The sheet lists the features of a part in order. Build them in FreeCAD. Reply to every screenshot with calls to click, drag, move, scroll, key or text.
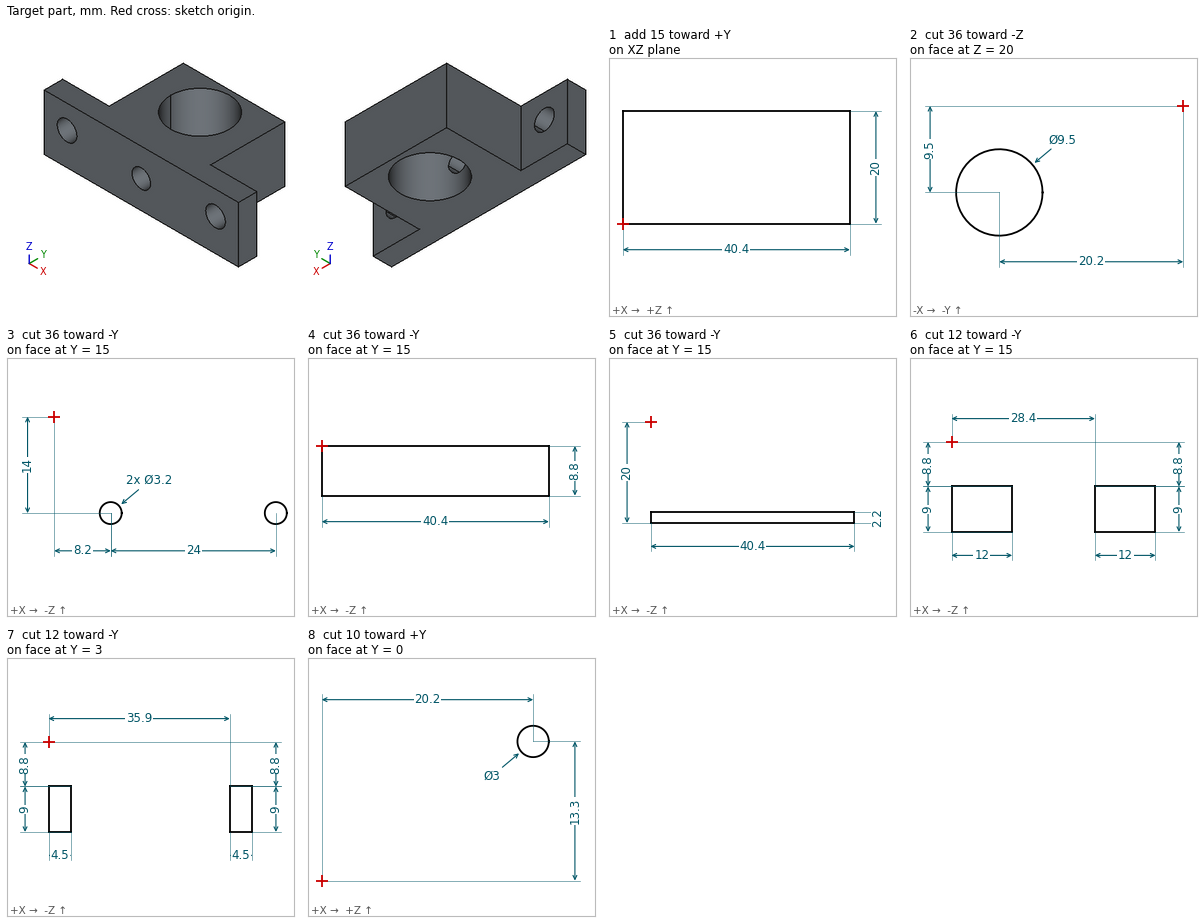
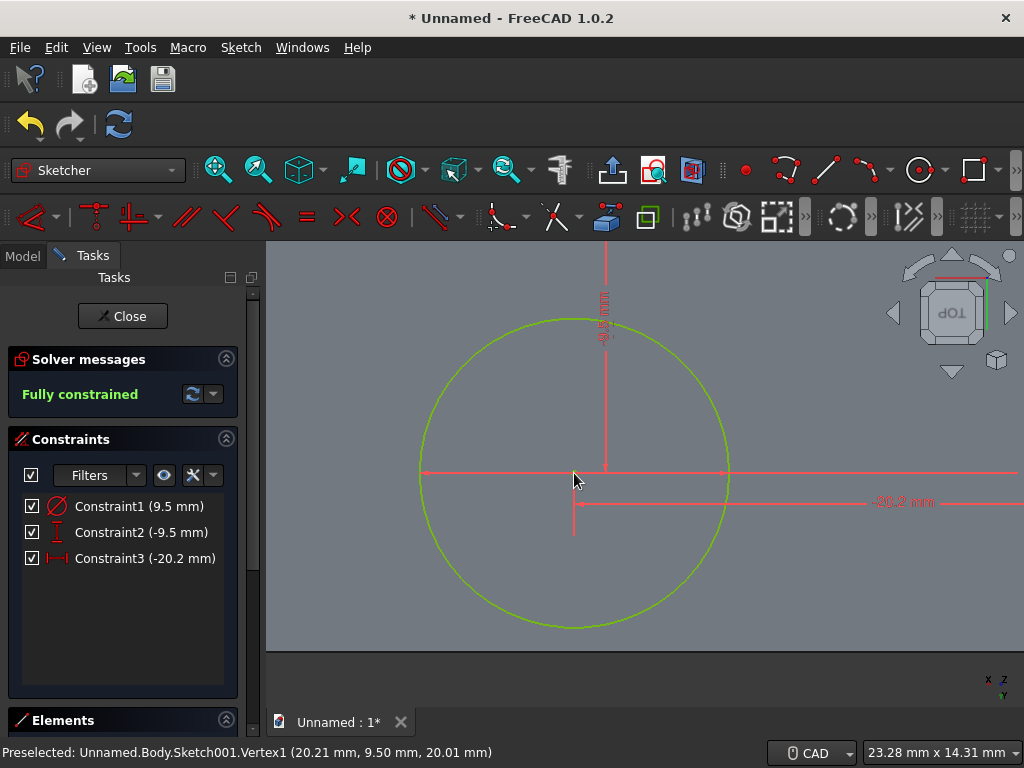
click(123, 316)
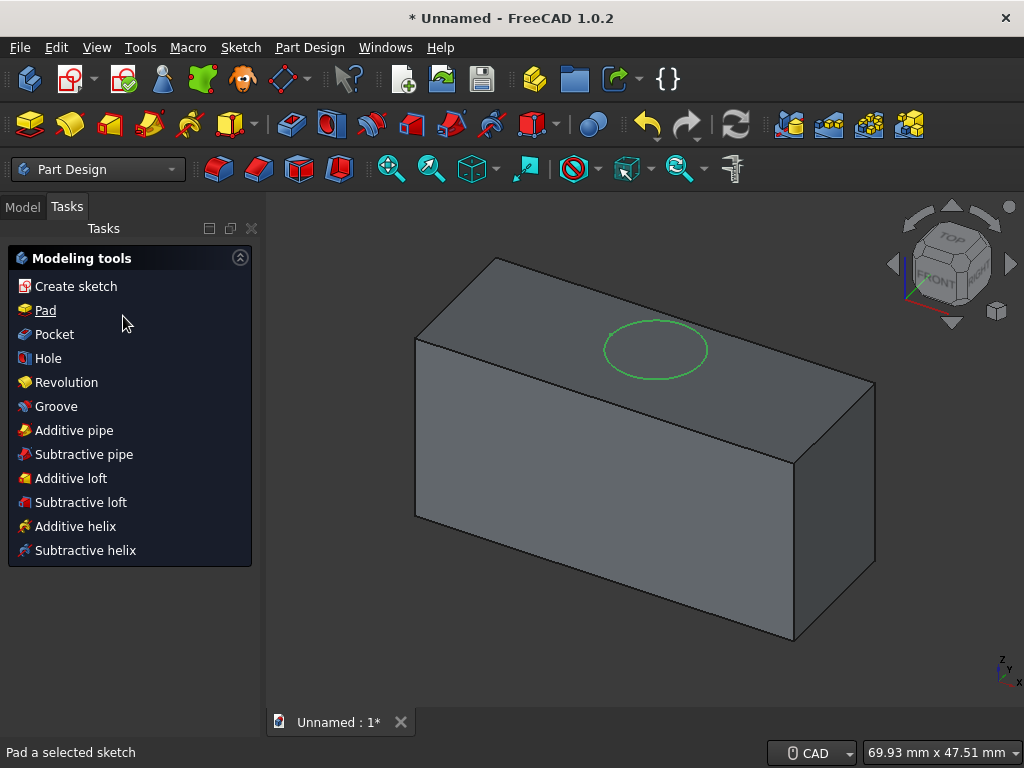
click(292, 124)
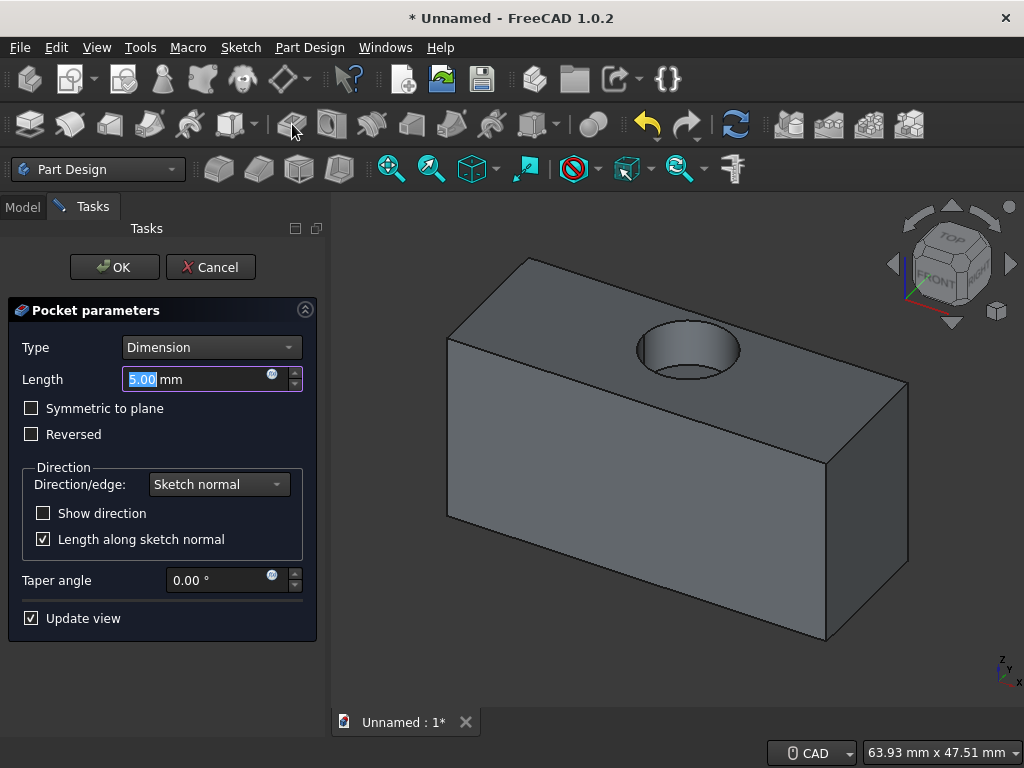
text(36)
key(Tab)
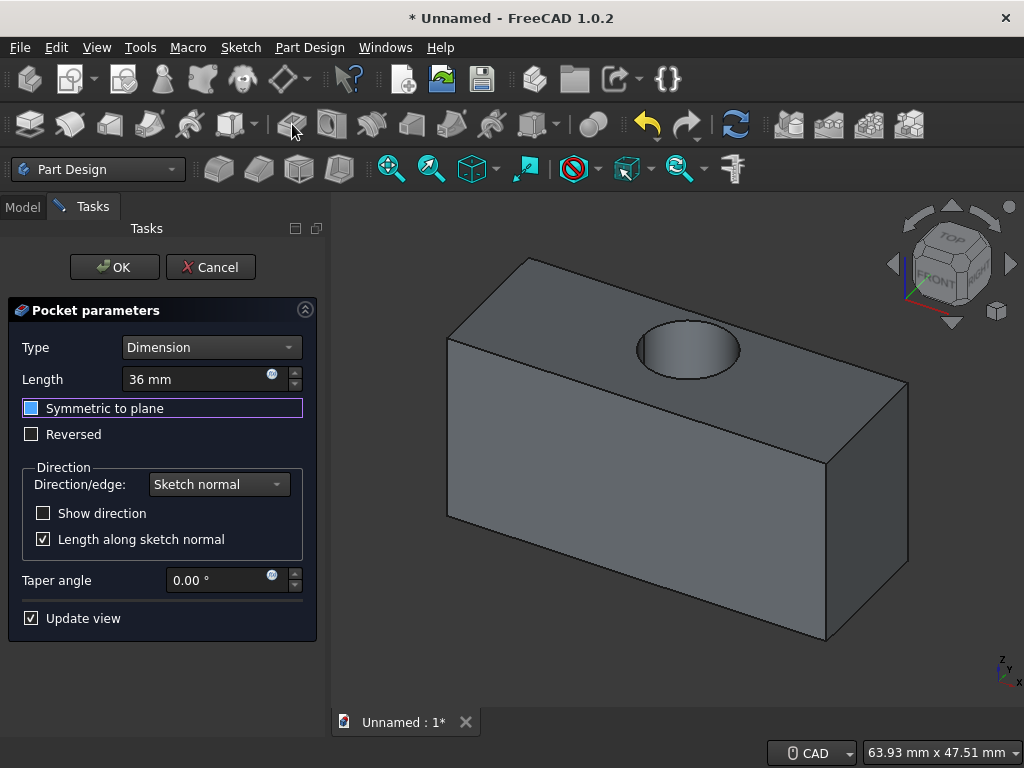
click(115, 267)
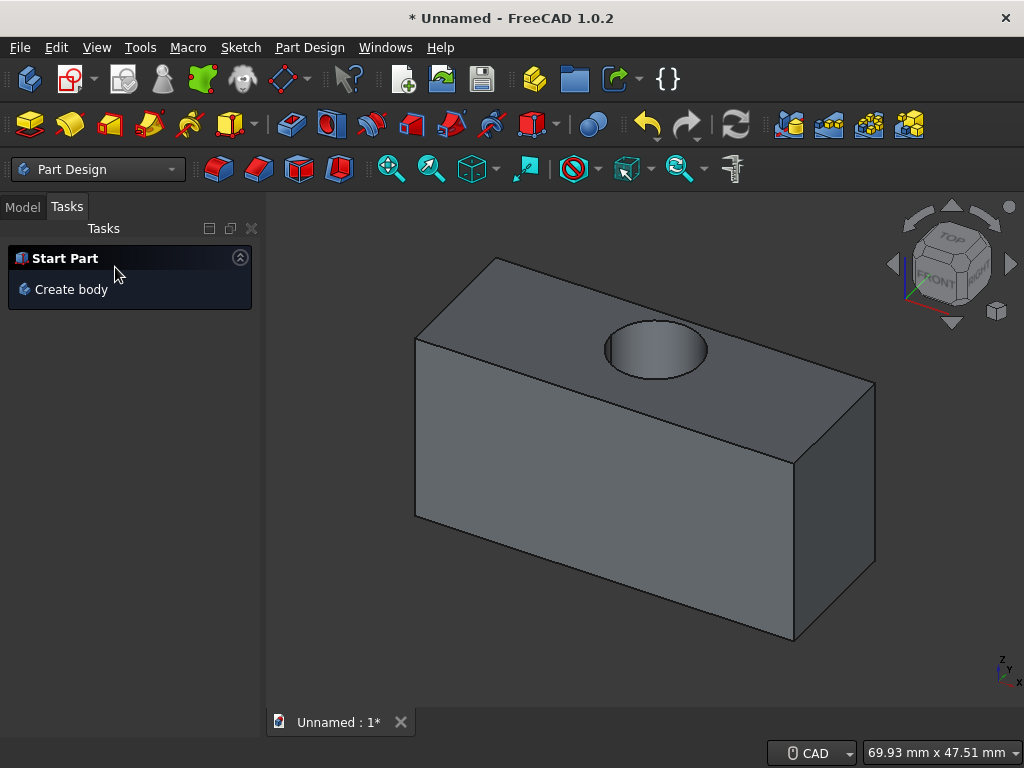
key(4)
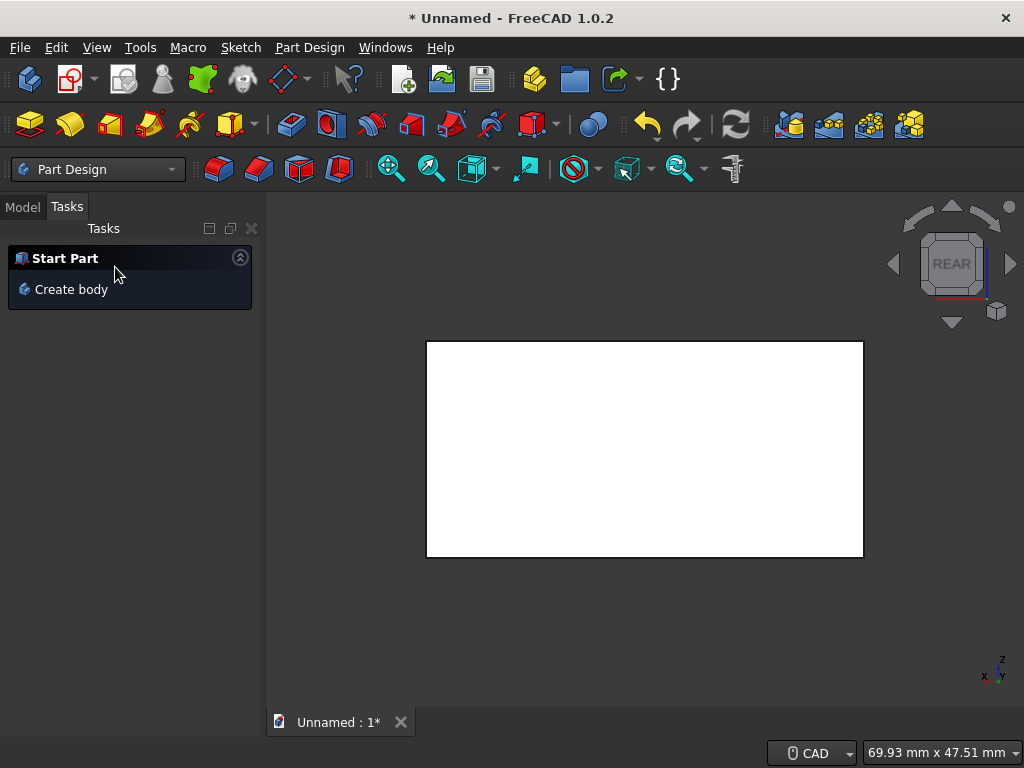
click(582, 449)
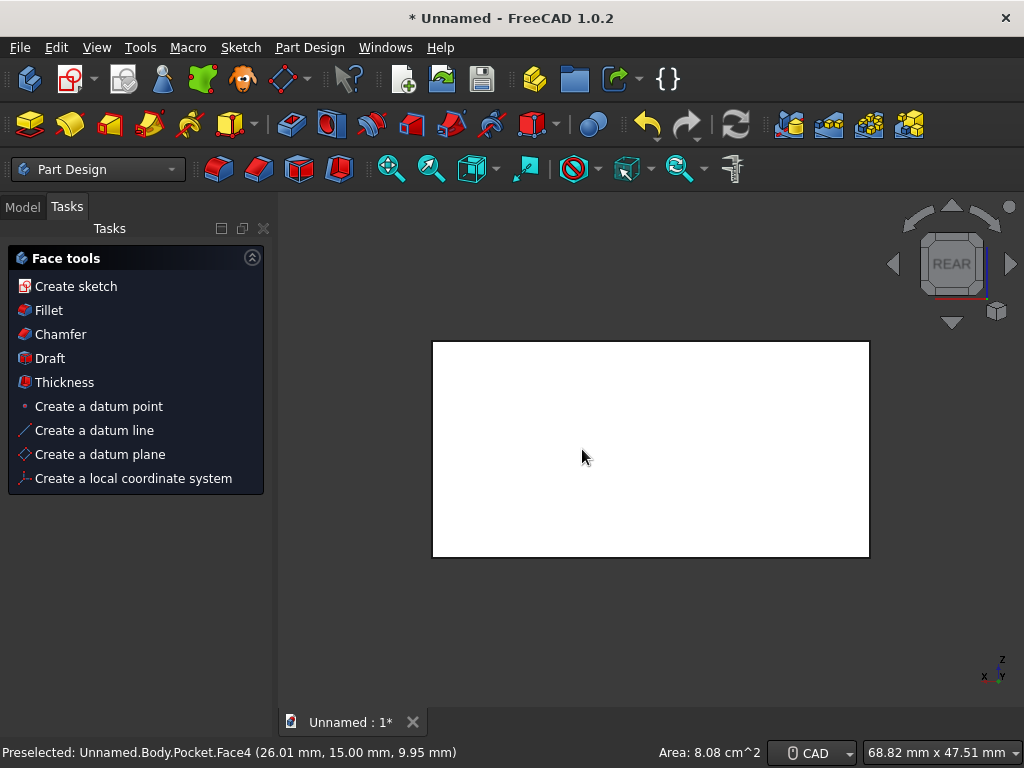
click(70, 80)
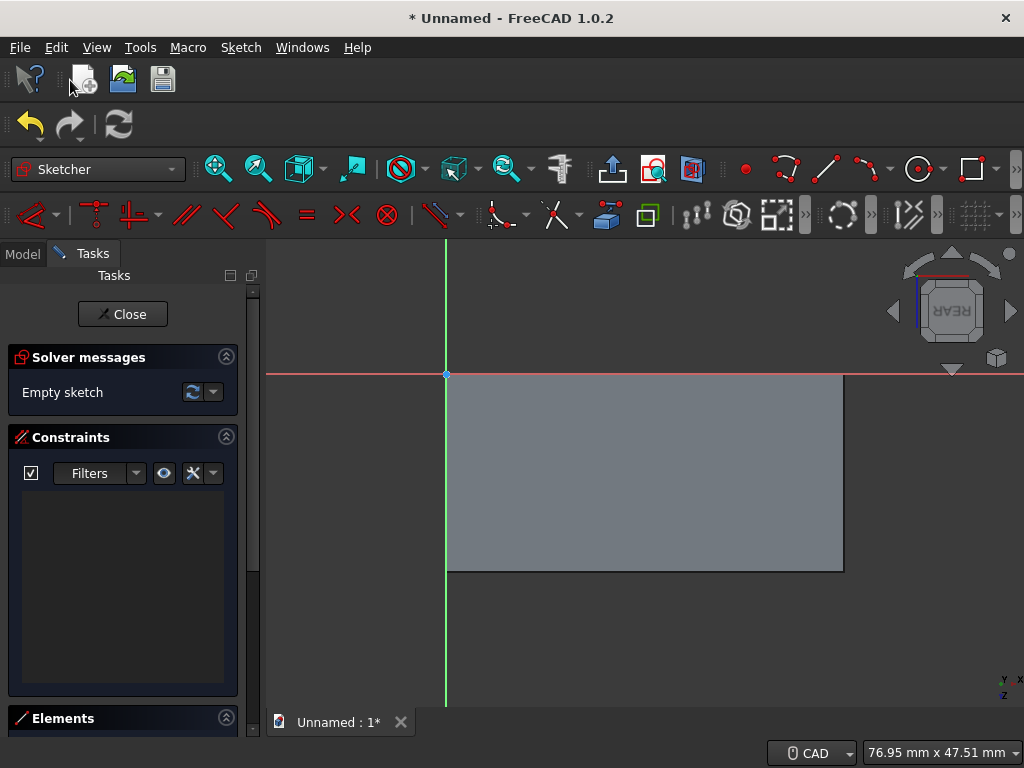
click(920, 170)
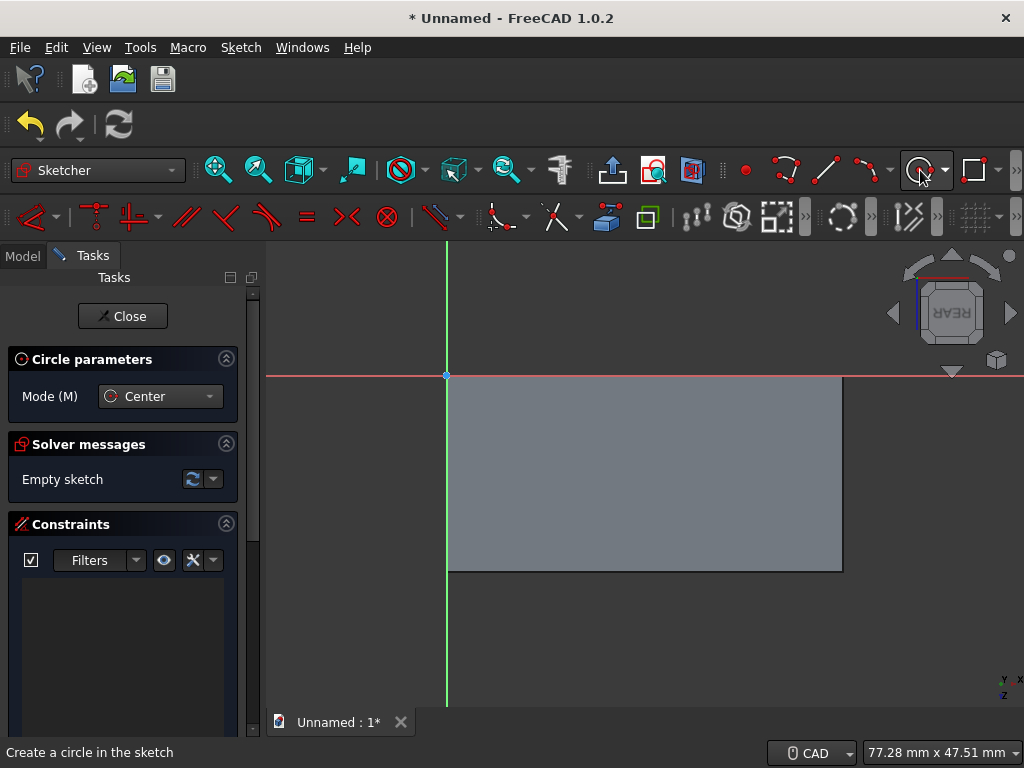
scroll(527, 513, up, 2)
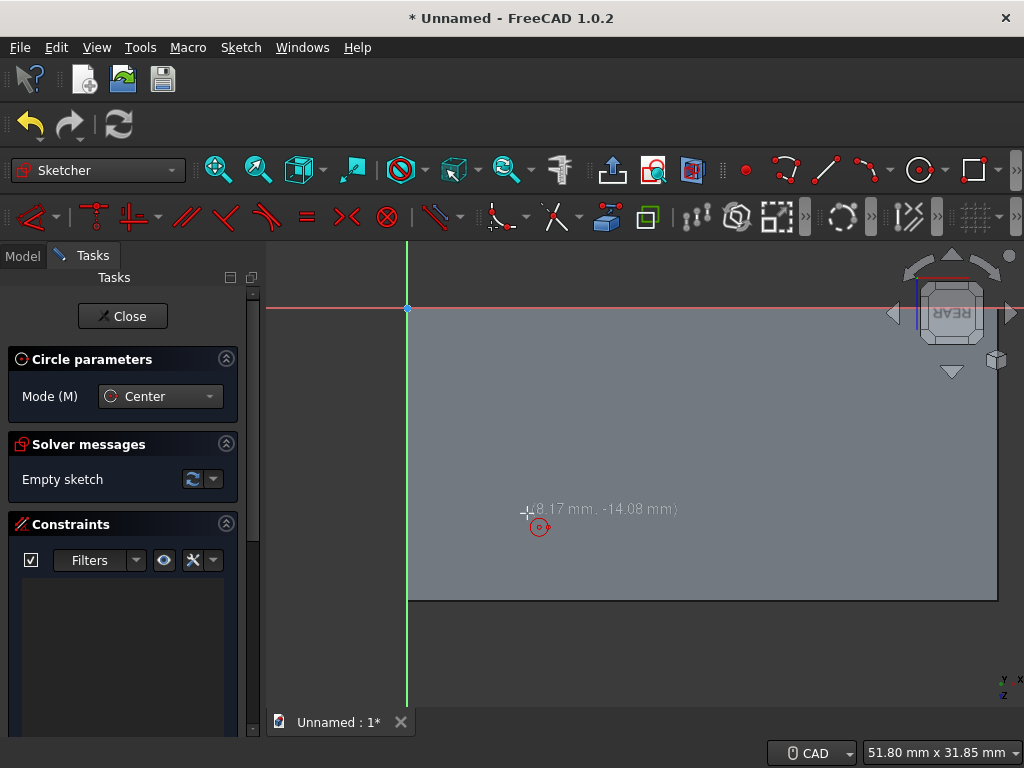
click(527, 513)
move(544, 497)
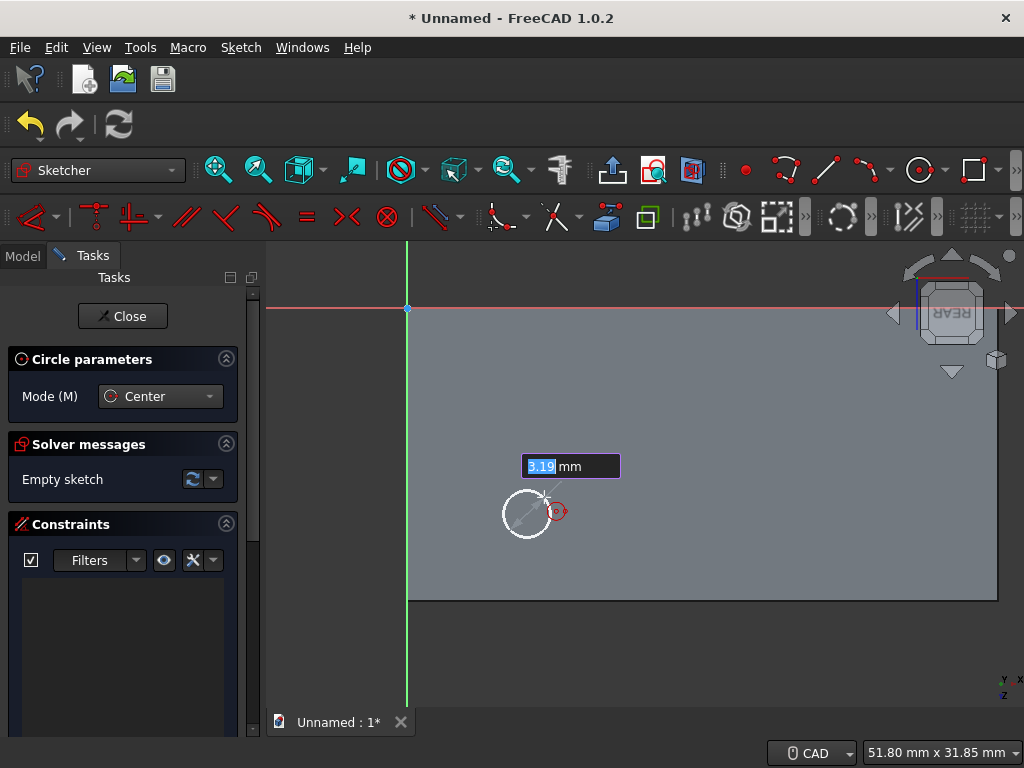
text(3.2)
key(Return)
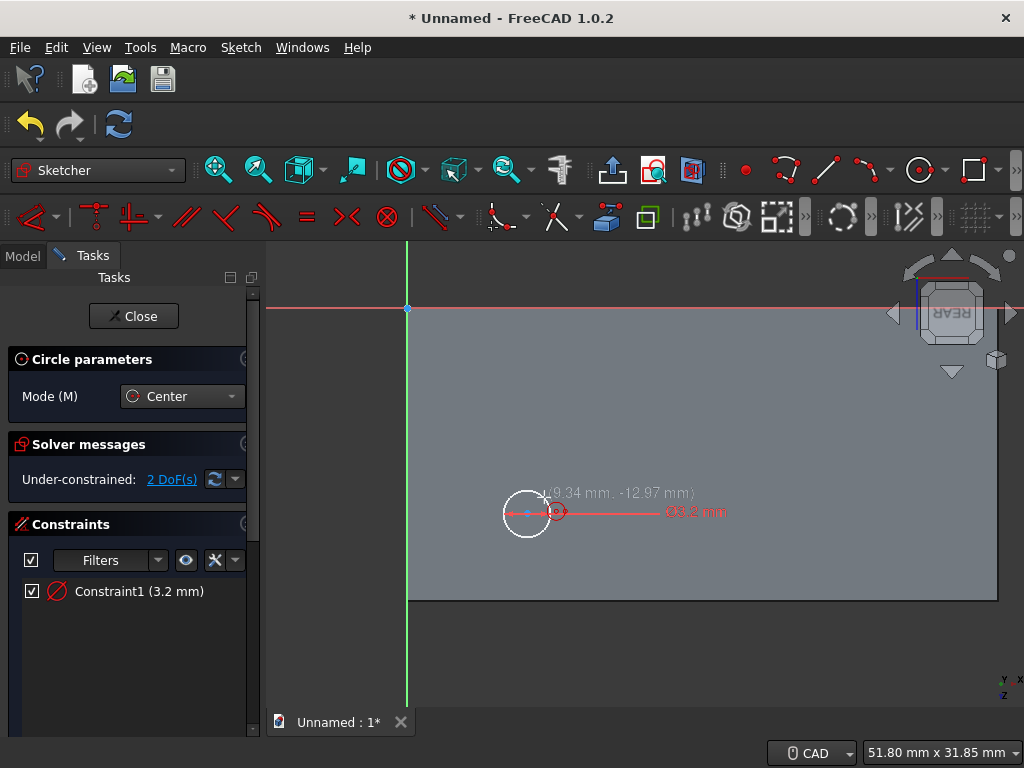
scroll(294, 679, down, 1)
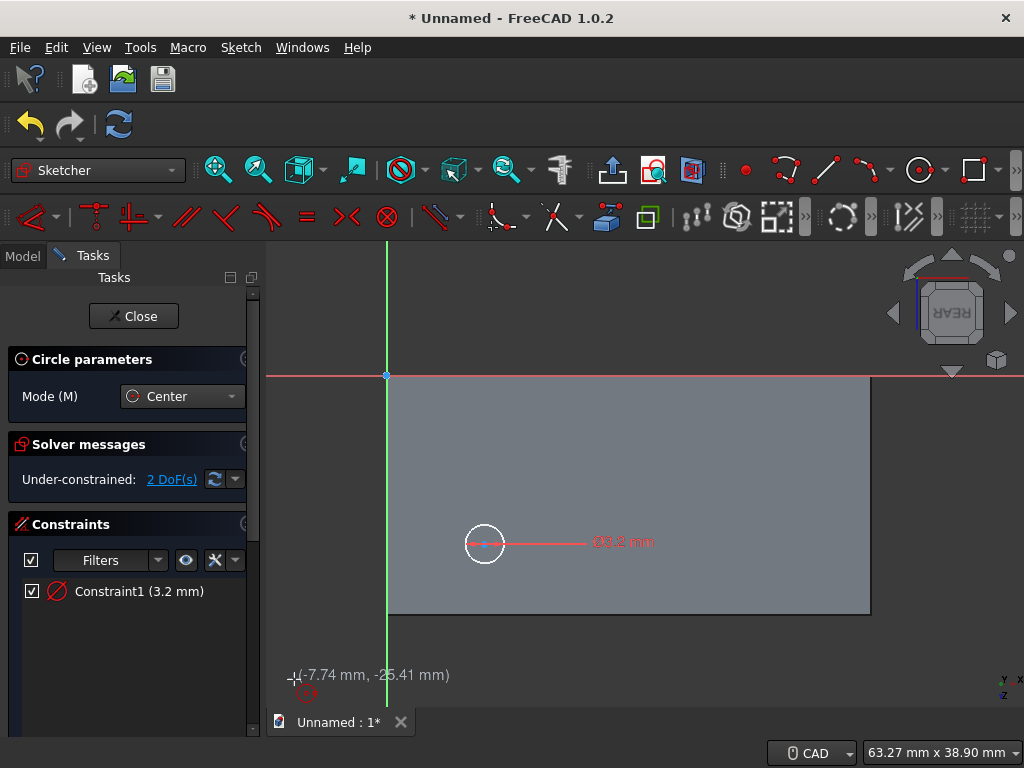
click(773, 543)
move(786, 530)